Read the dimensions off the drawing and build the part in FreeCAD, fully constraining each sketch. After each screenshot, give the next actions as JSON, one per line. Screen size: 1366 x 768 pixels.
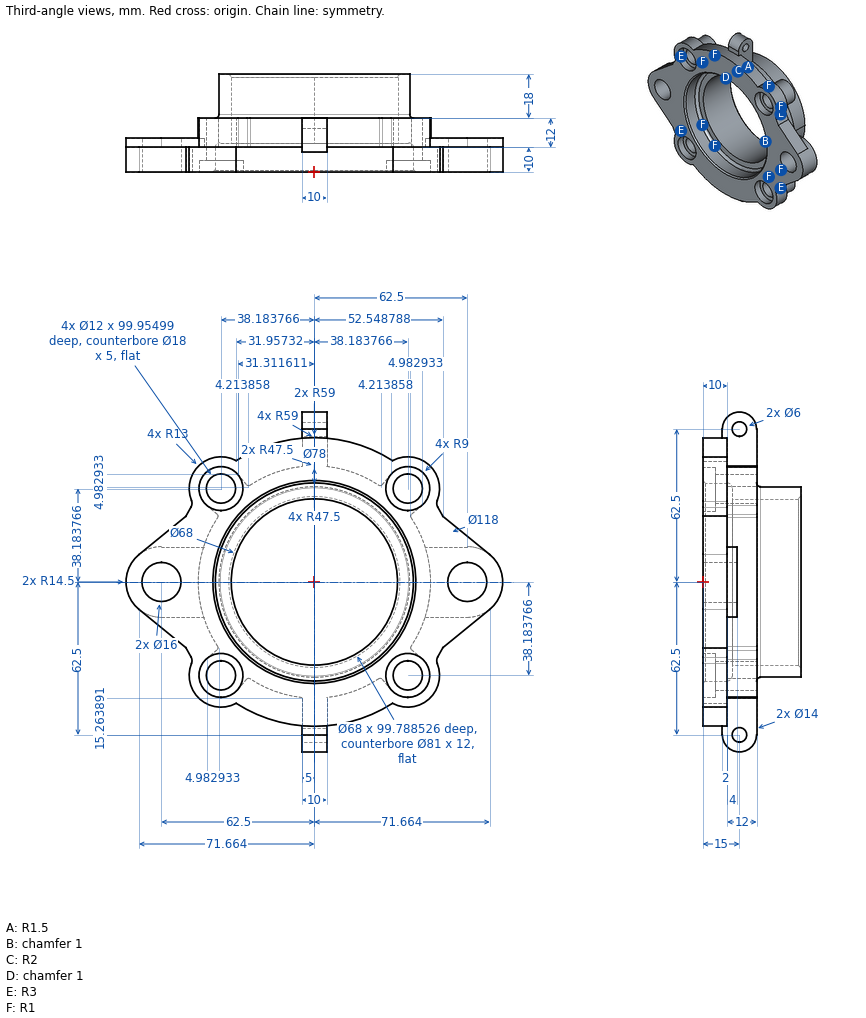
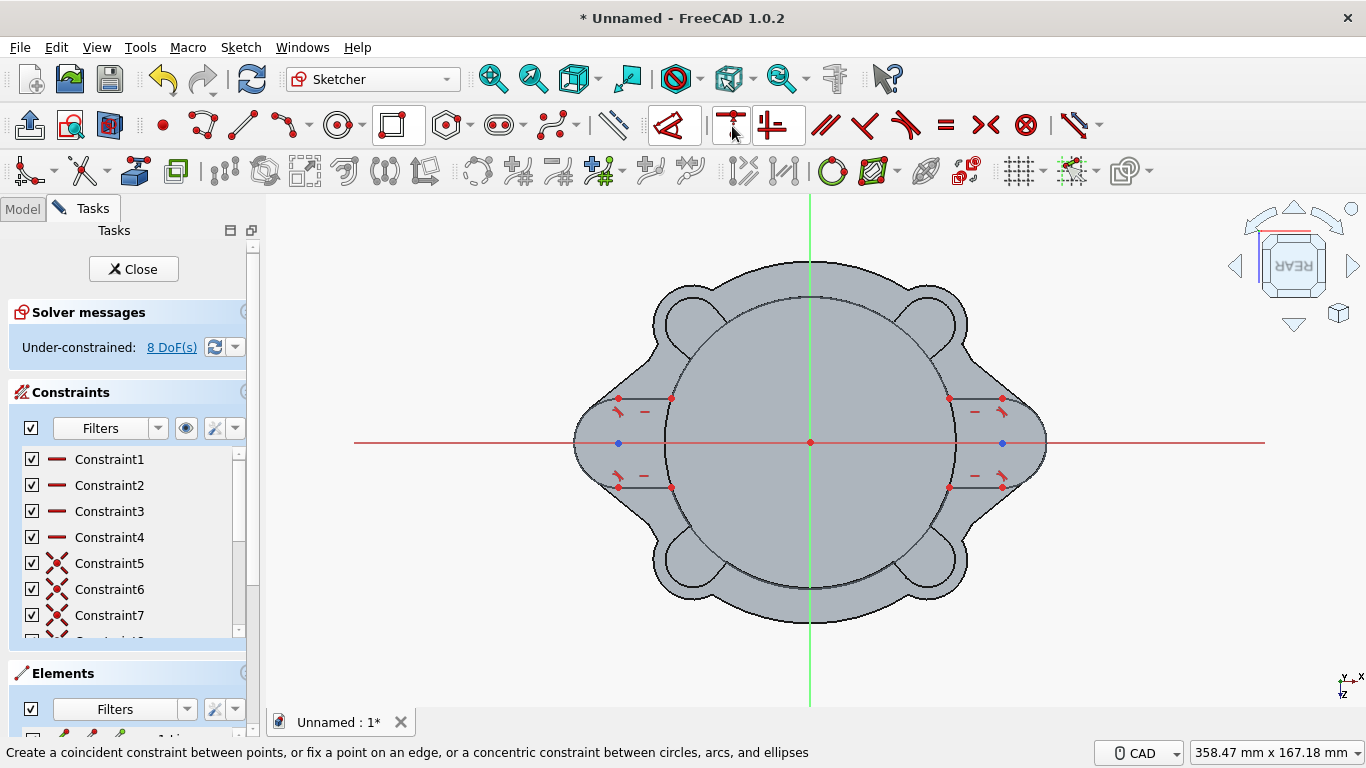
{"action": "left_click", "coordinate": [583, 417]}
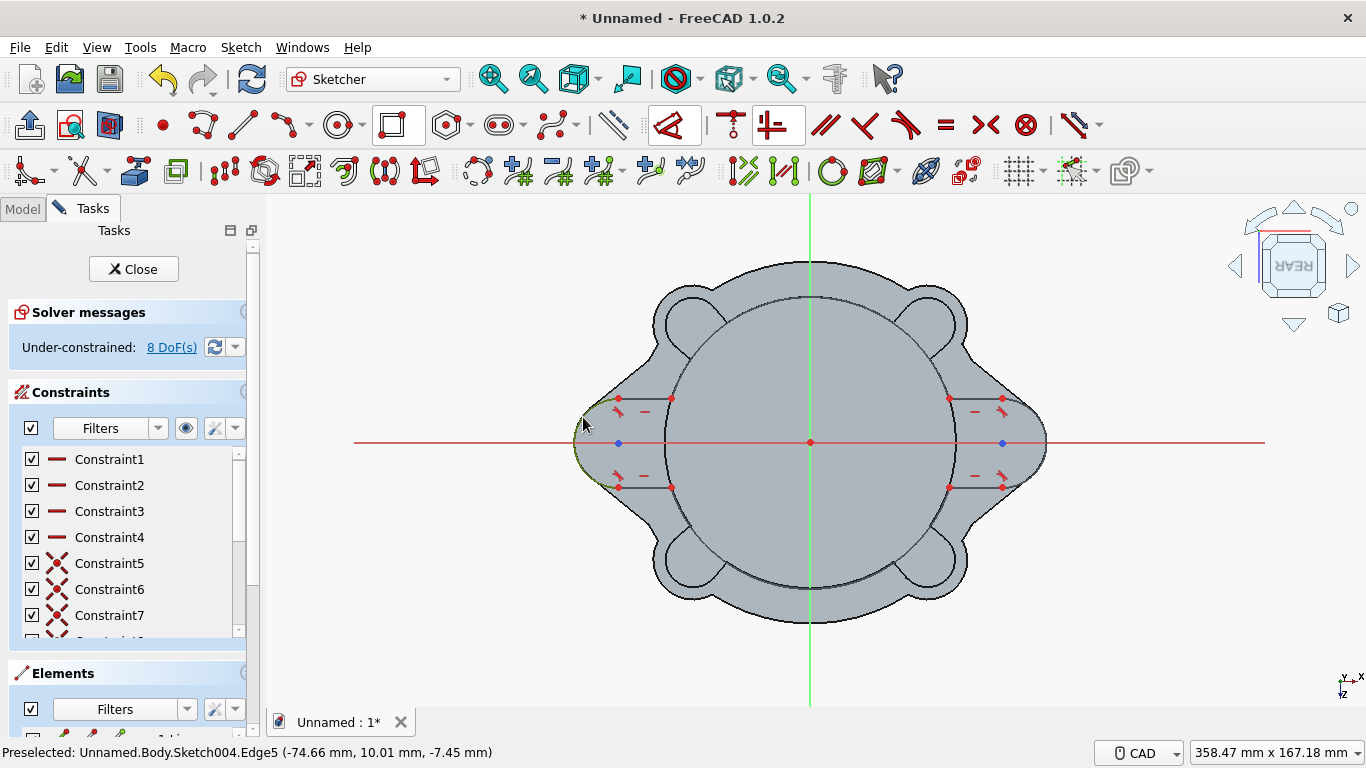
{"action": "left_click", "coordinate": [1038, 470]}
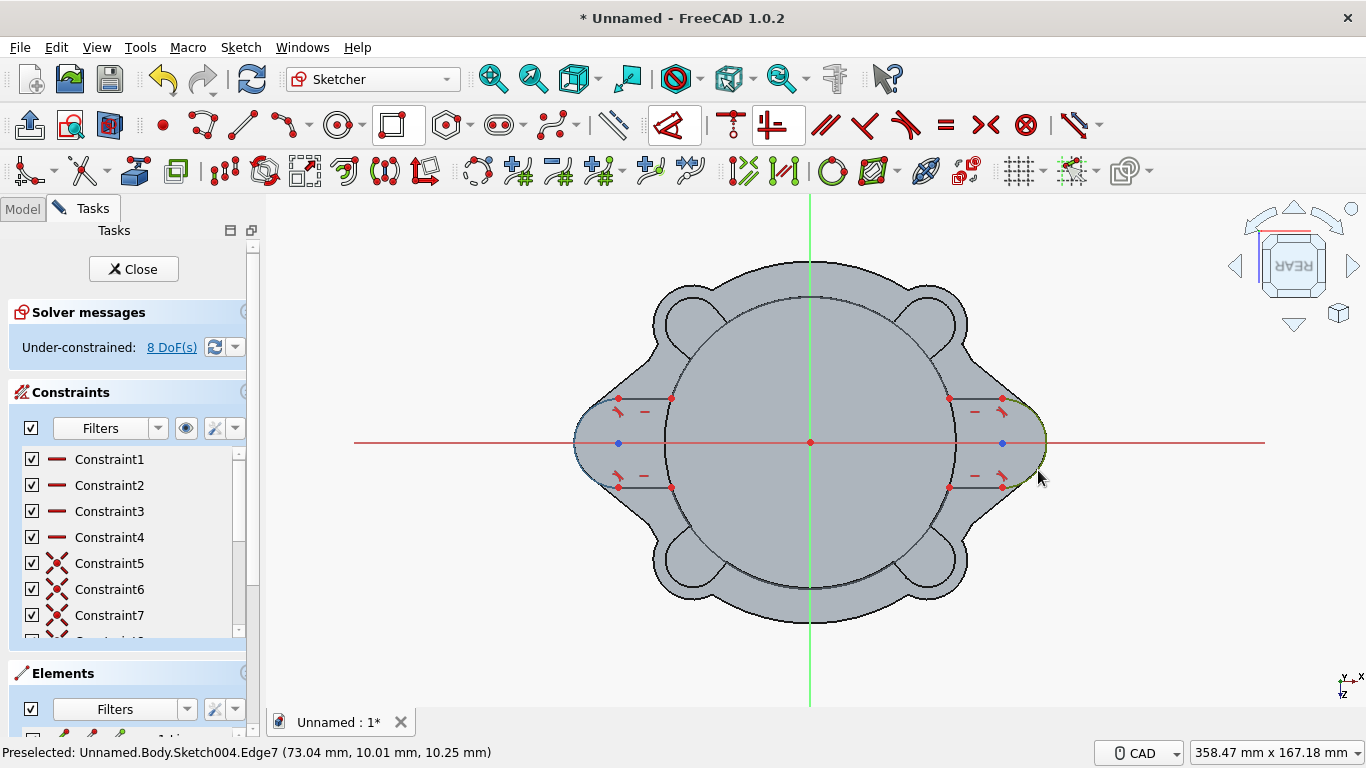
{"action": "left_click", "coordinate": [946, 126]}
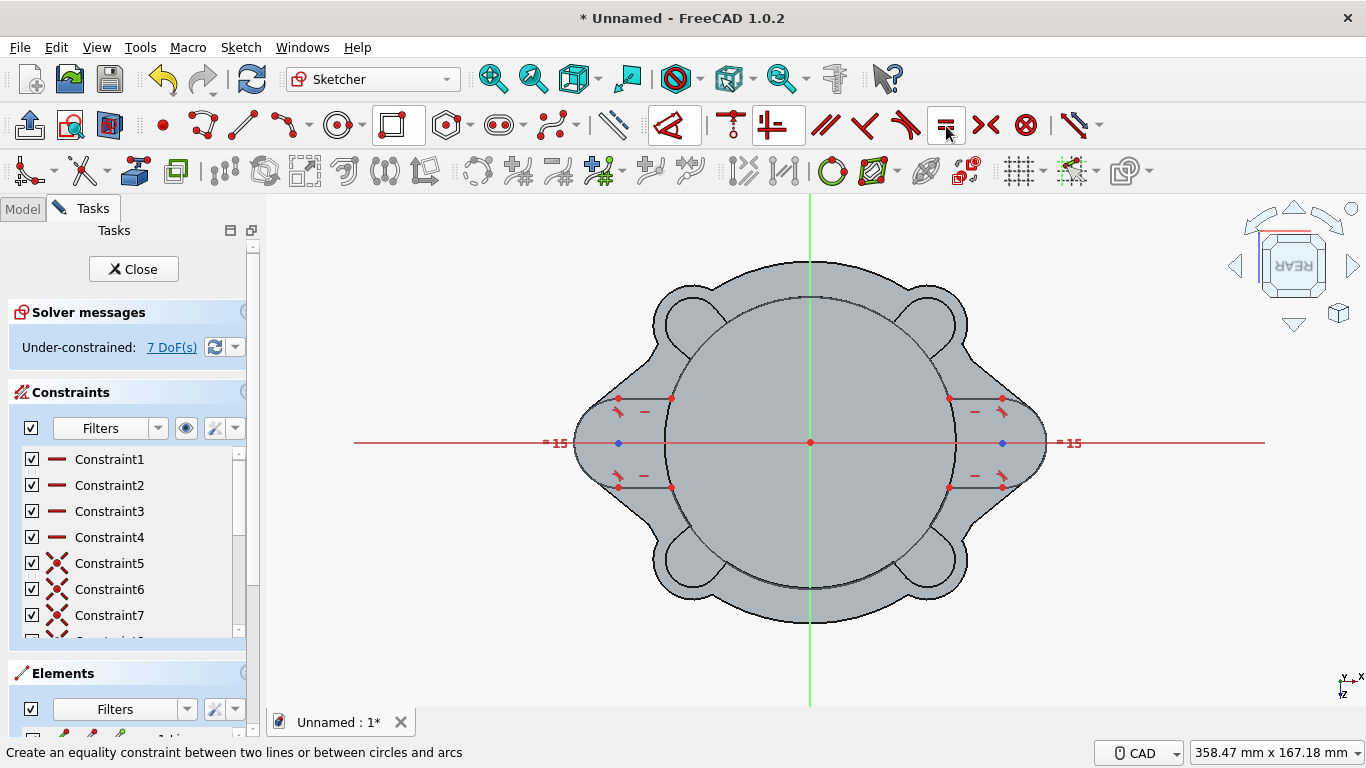
{"action": "left_click", "coordinate": [740, 571]}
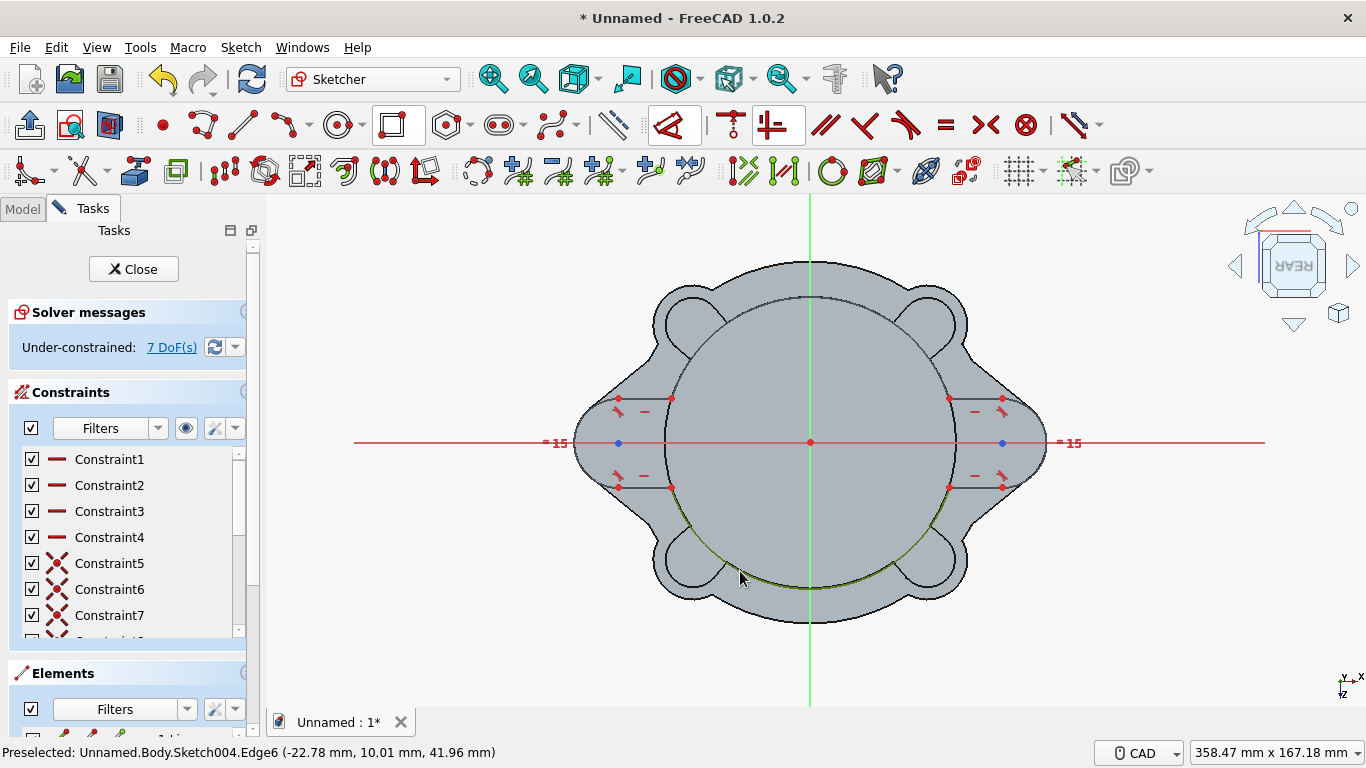
{"action": "left_click", "coordinate": [881, 315]}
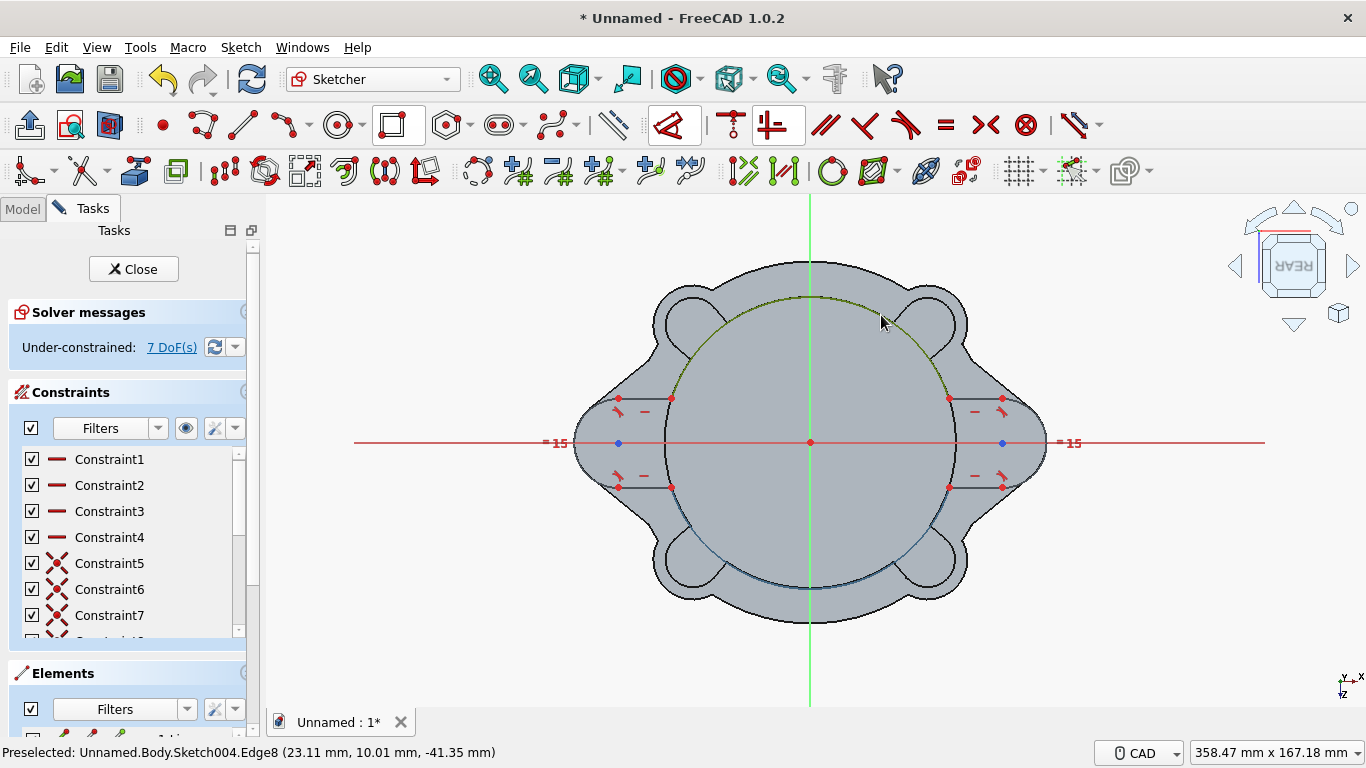
{"action": "left_click", "coordinate": [946, 126]}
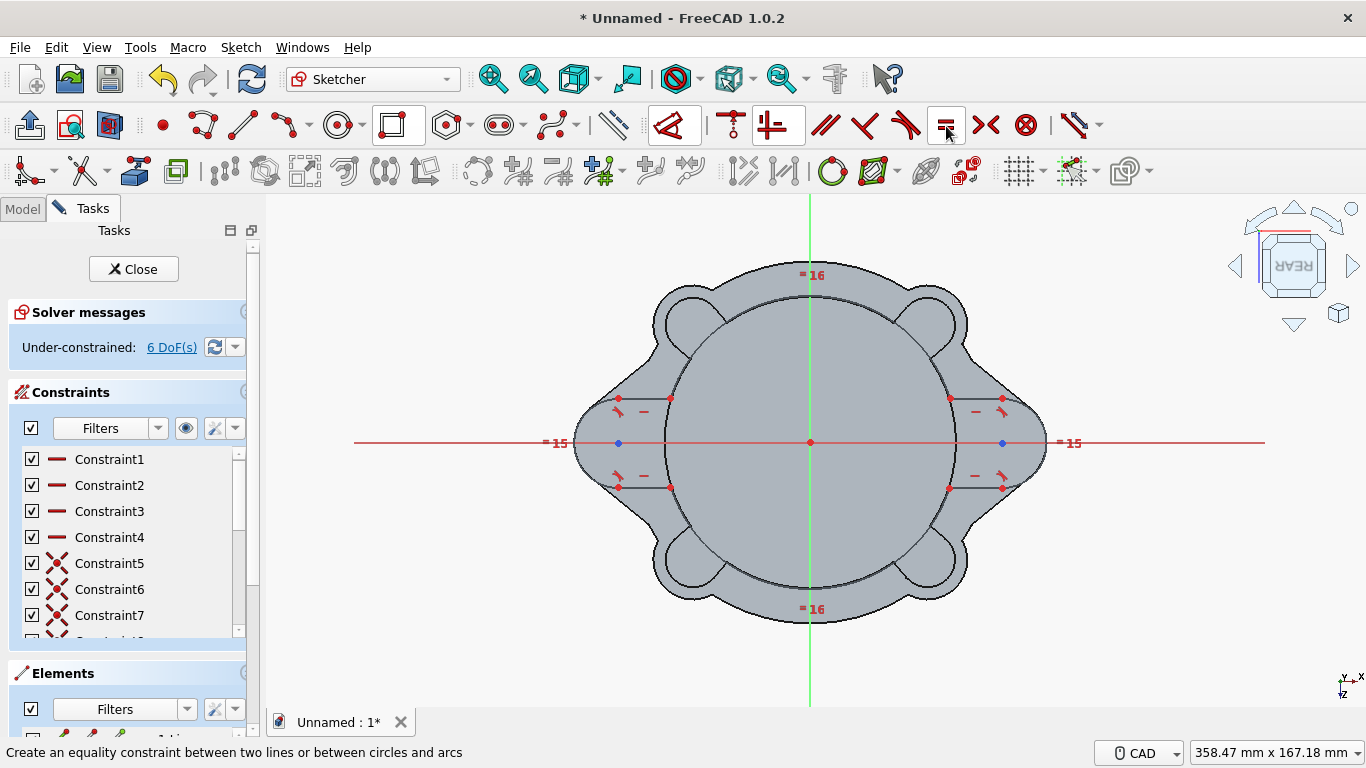
{"action": "left_click", "coordinate": [619, 443]}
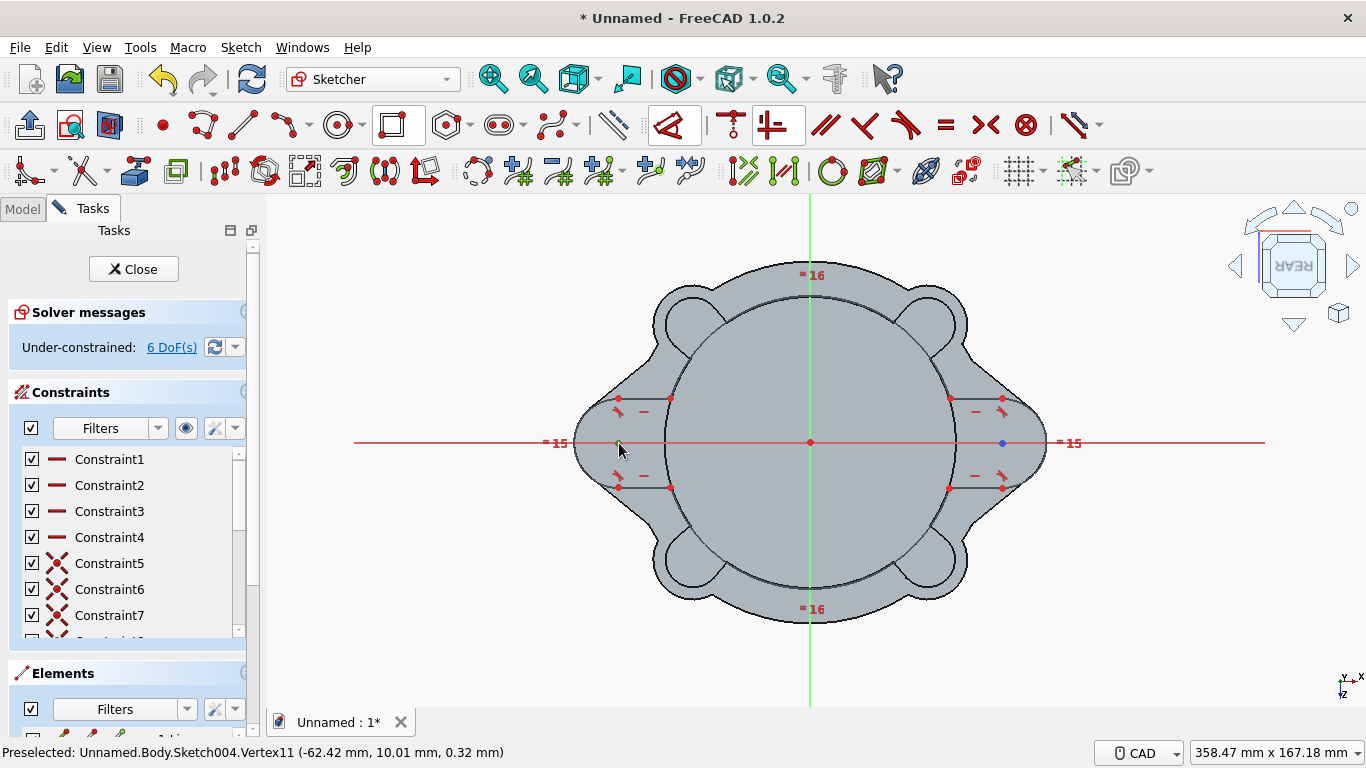
{"action": "left_click", "coordinate": [359, 443]}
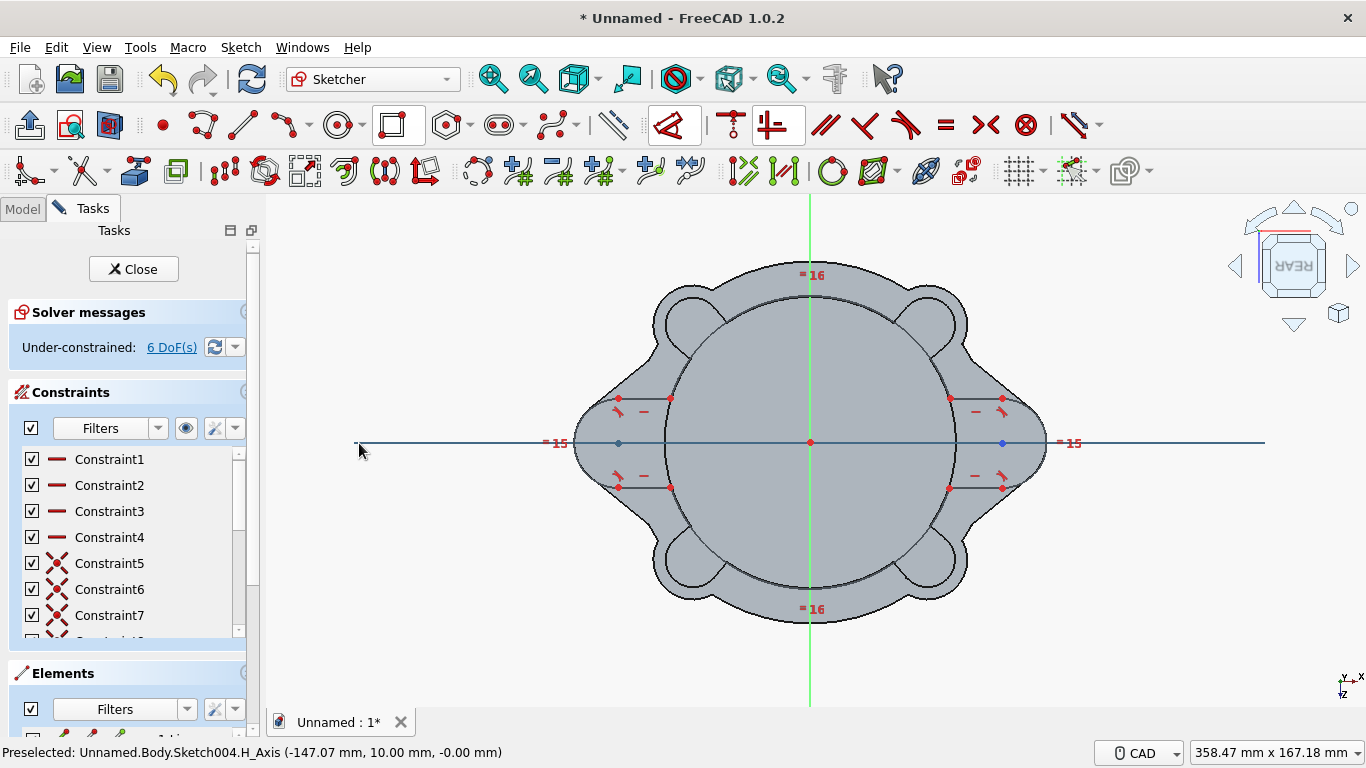
{"action": "left_click", "coordinate": [732, 126]}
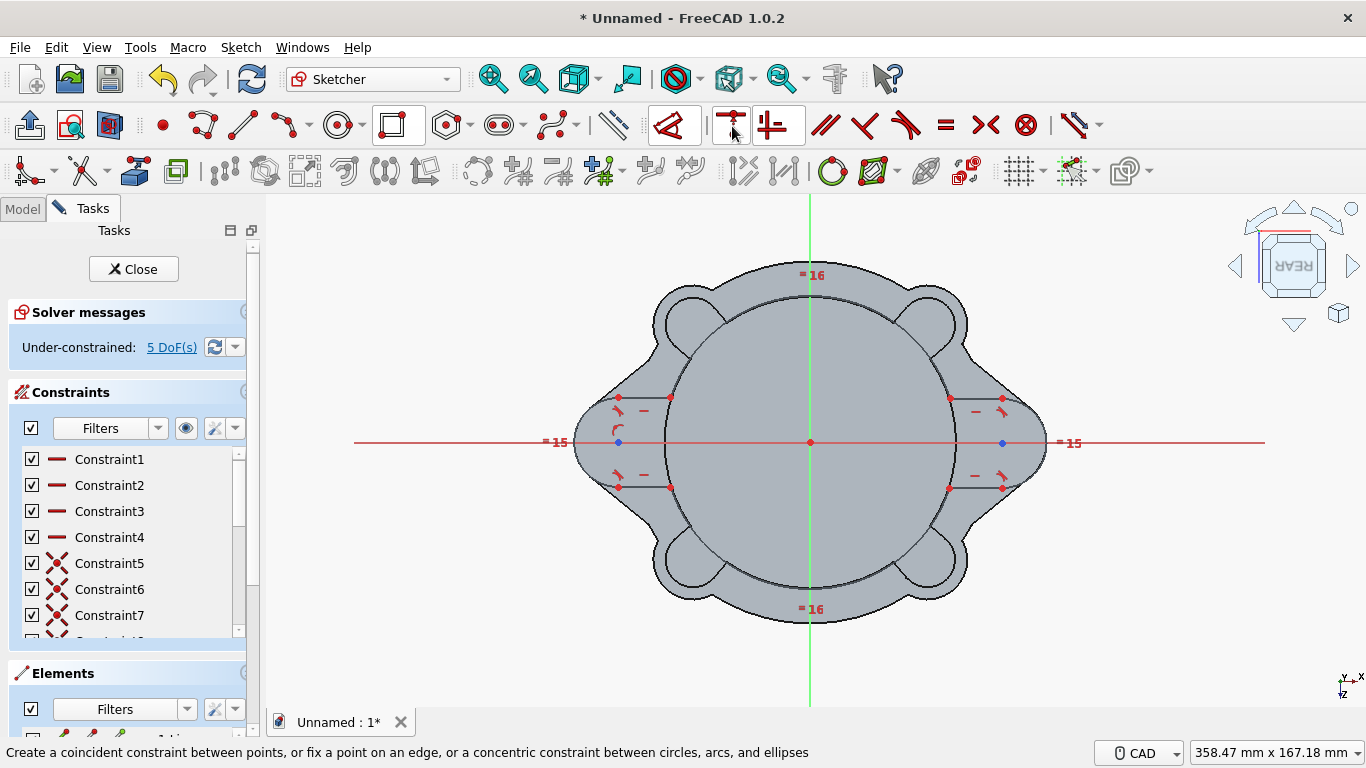
{"action": "left_click", "coordinate": [1002, 443]}